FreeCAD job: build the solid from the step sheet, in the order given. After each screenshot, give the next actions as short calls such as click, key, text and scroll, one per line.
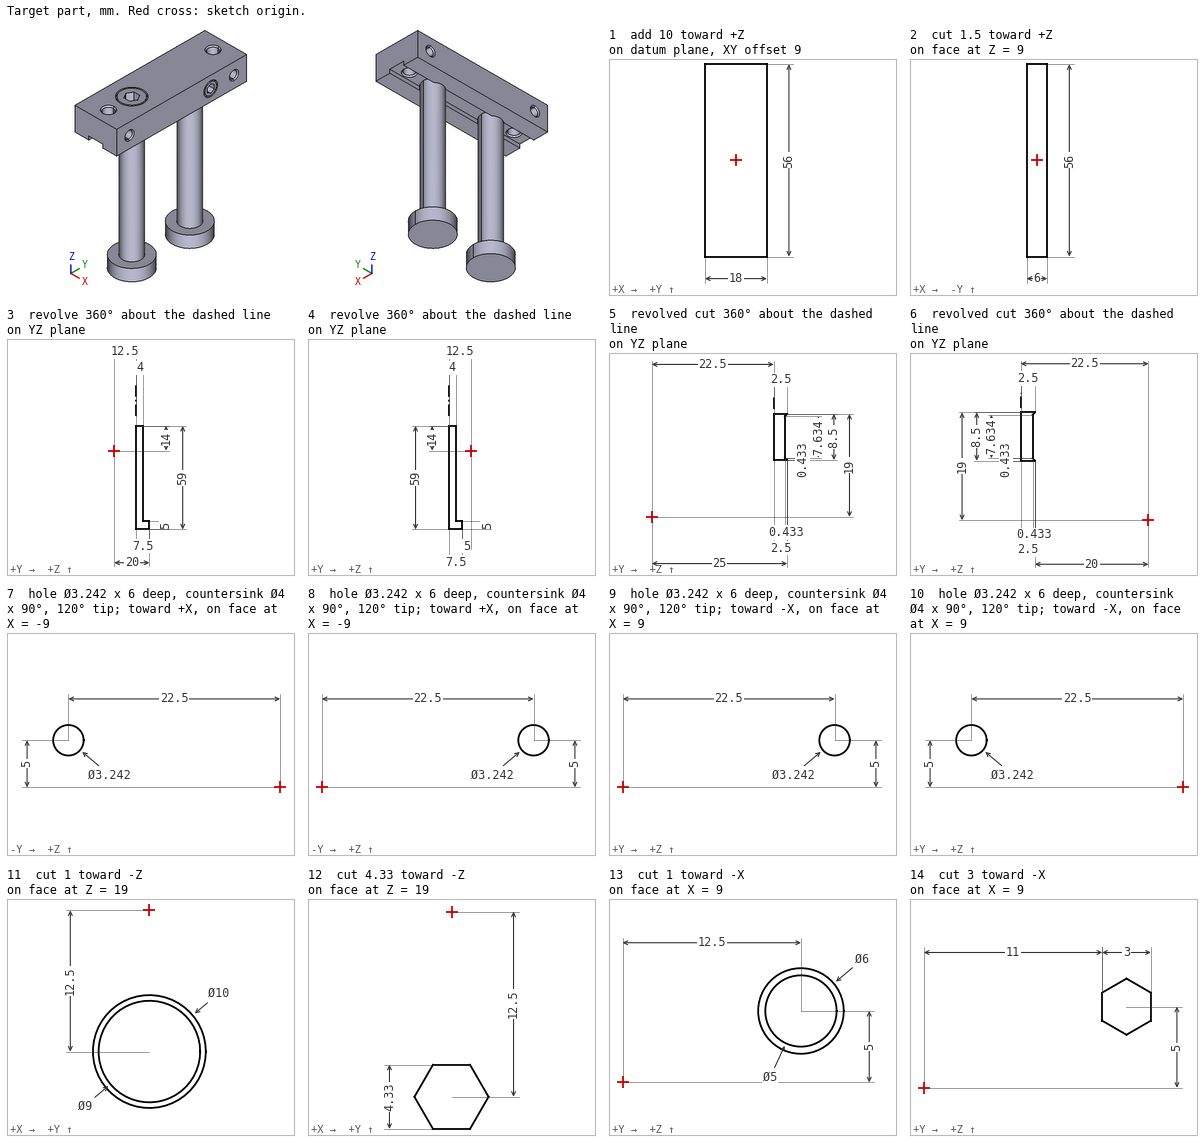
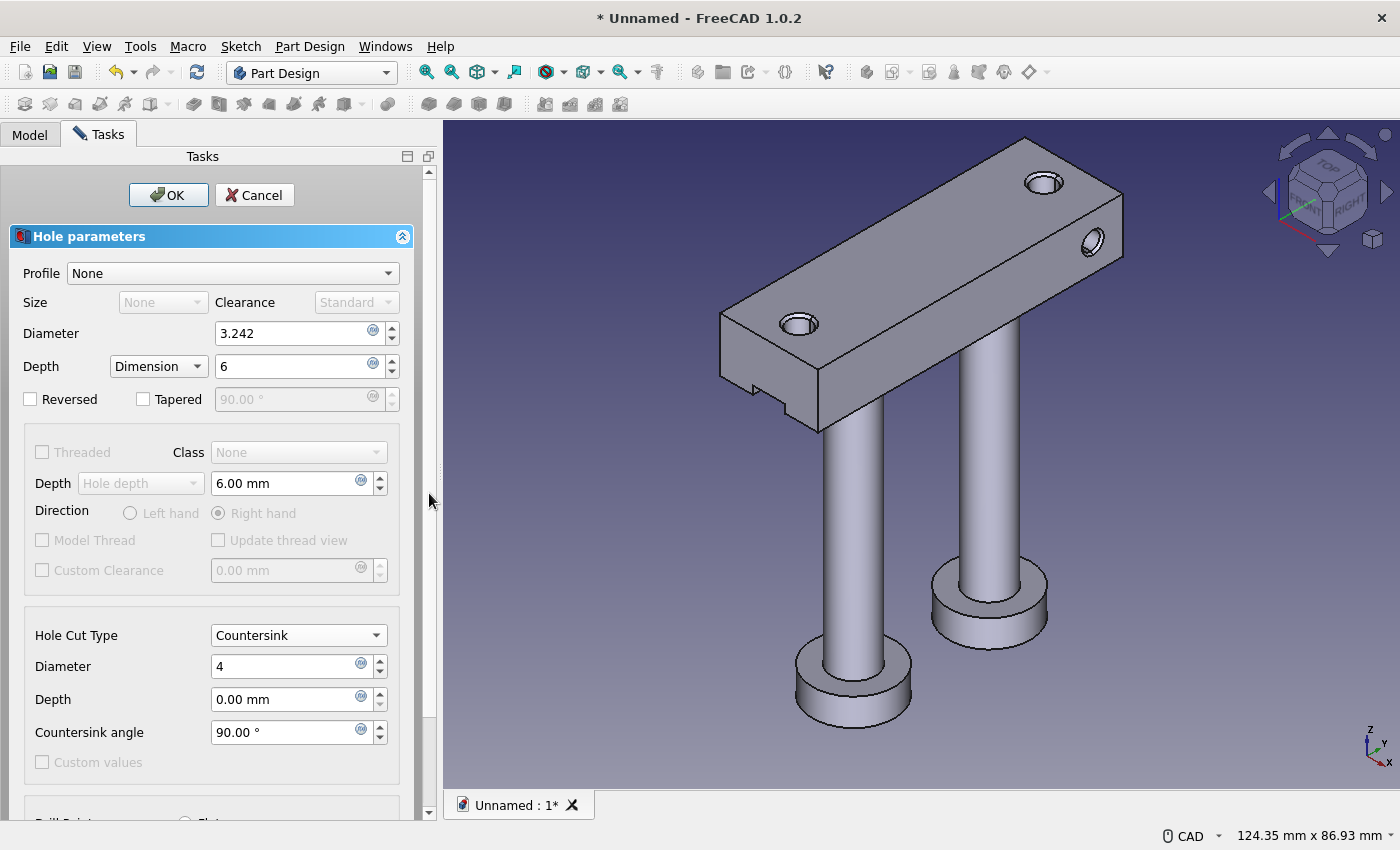
click(169, 195)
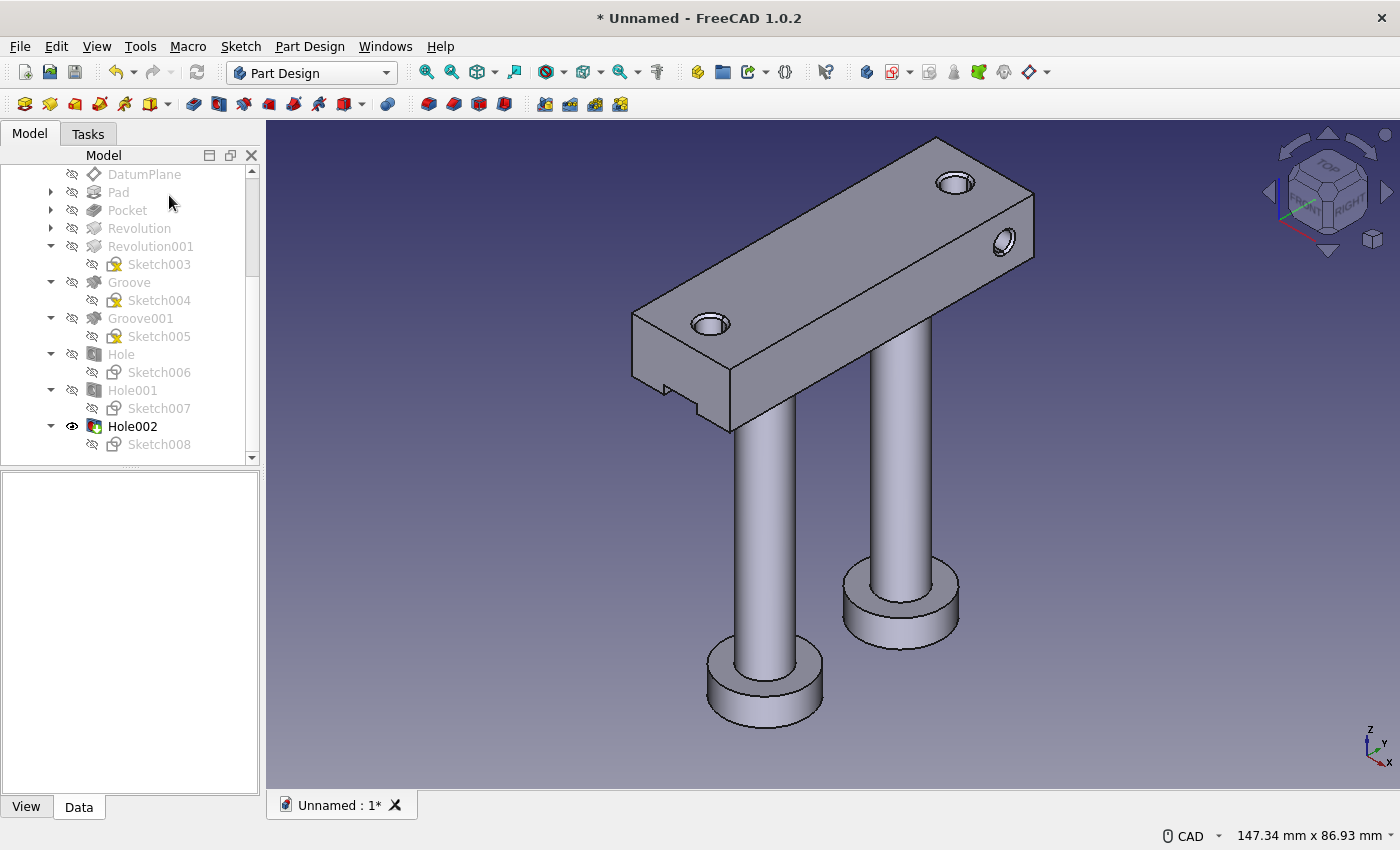
click(926, 287)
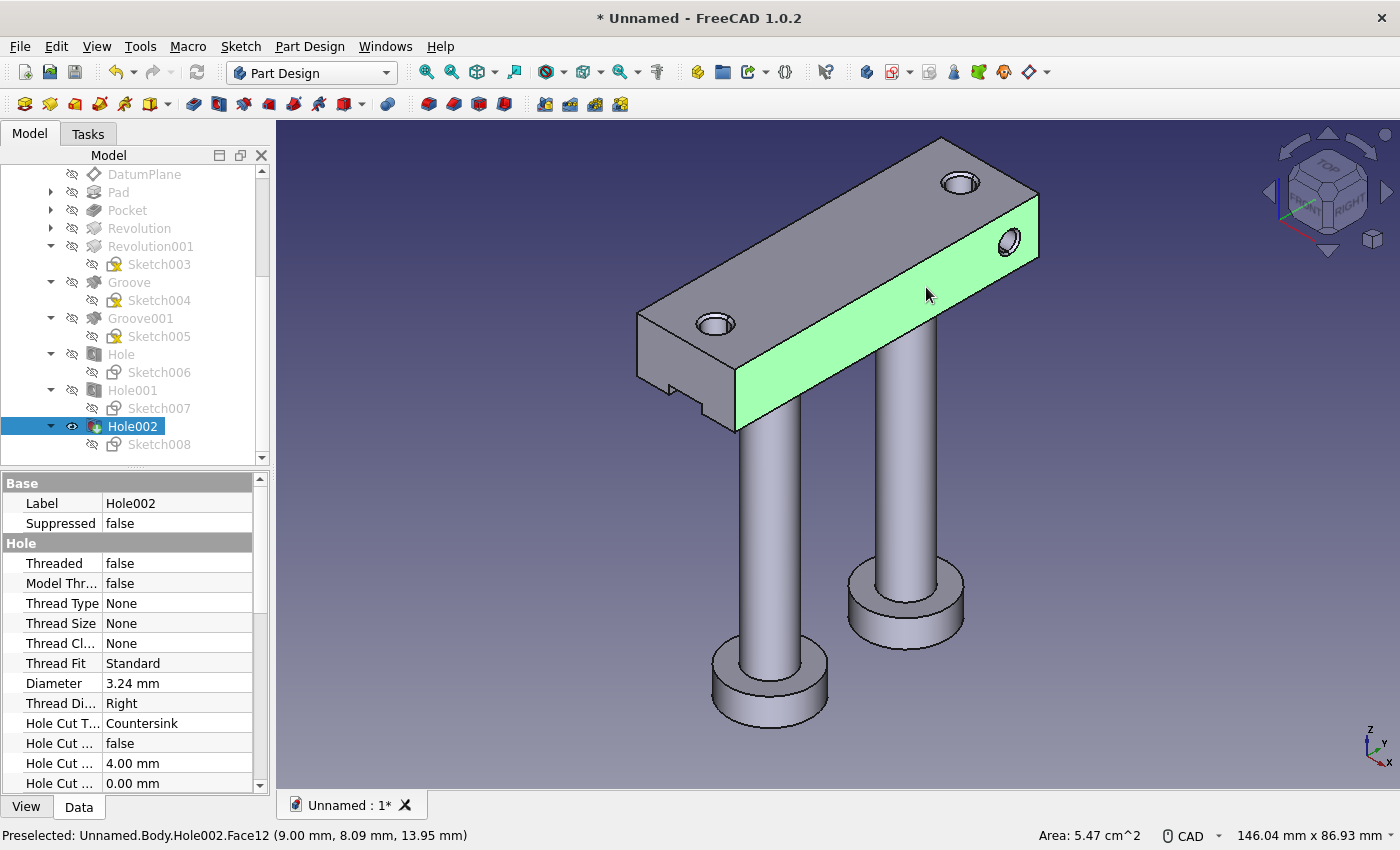
click(892, 72)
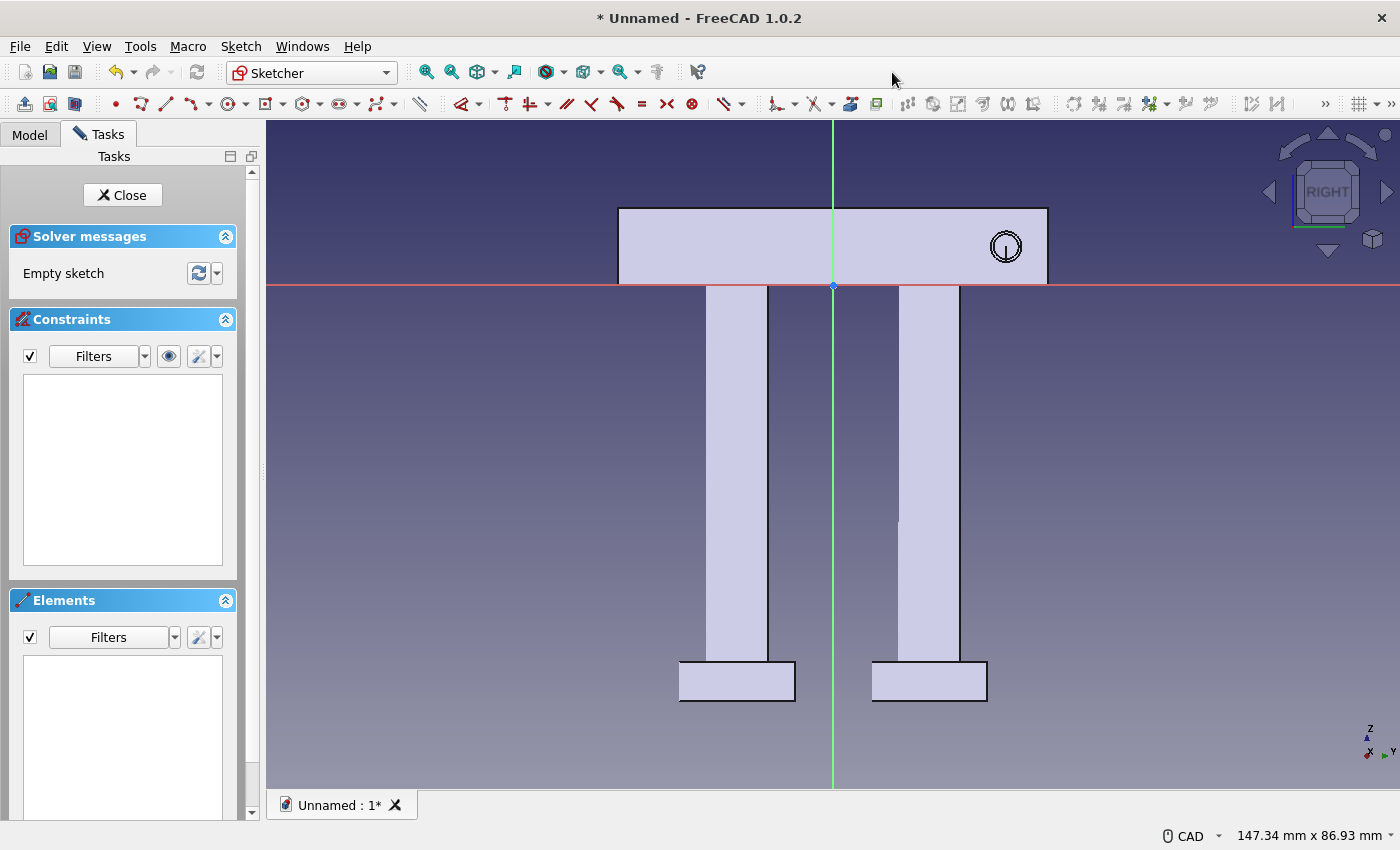
scroll(653, 233, up, 14)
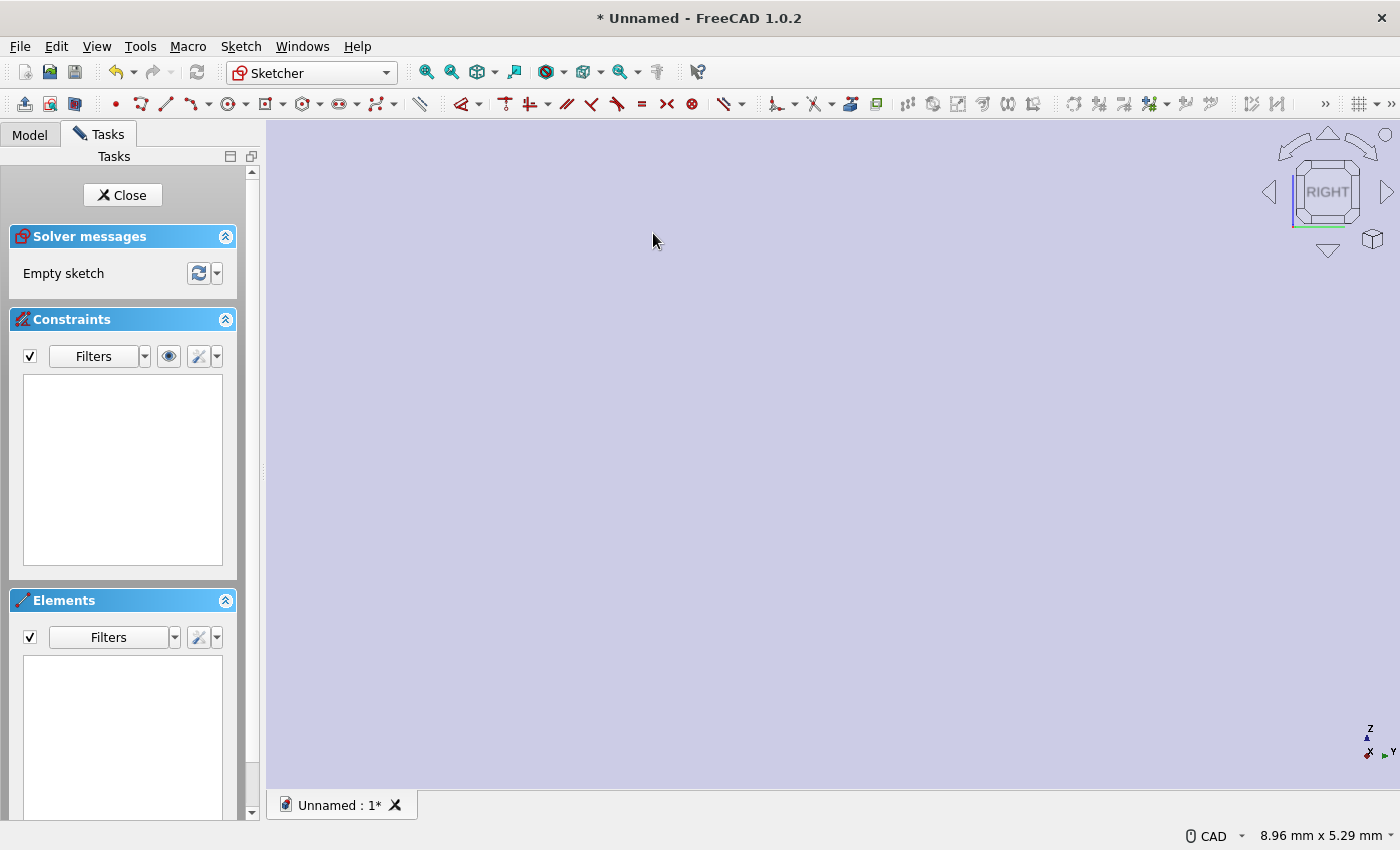
click(228, 104)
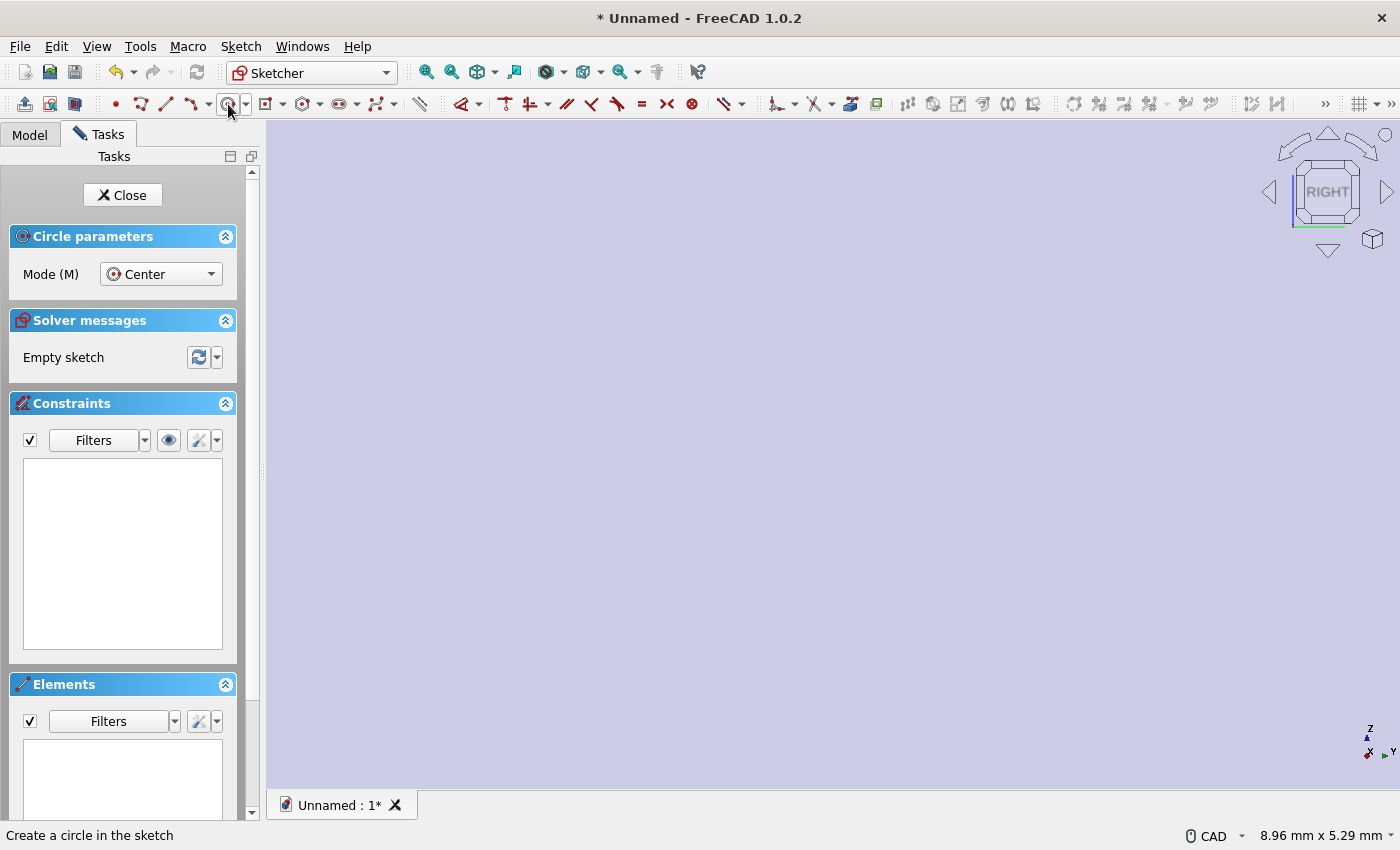
click(760, 456)
move(905, 311)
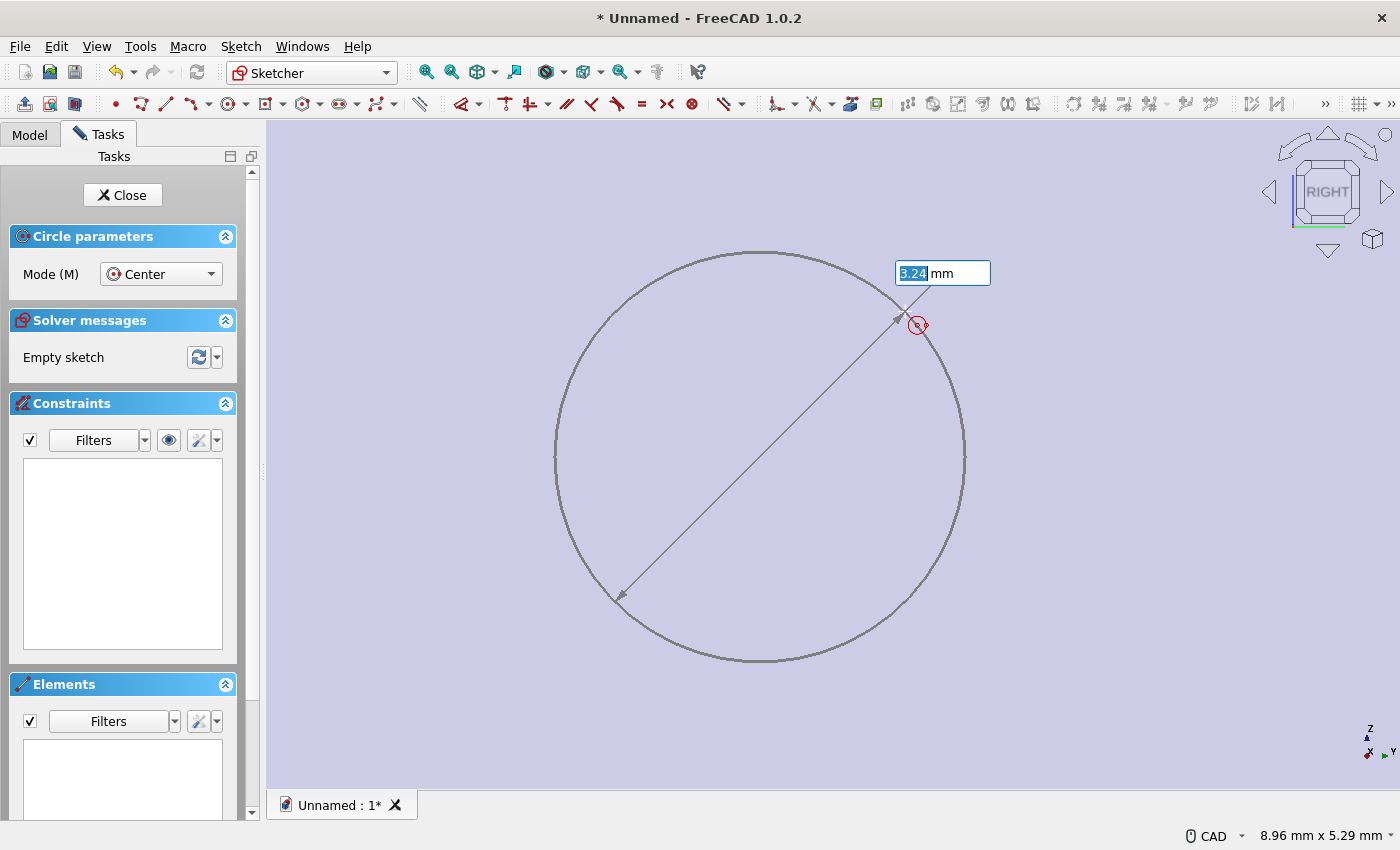
text(3.242)
key(Return)
key(Escape)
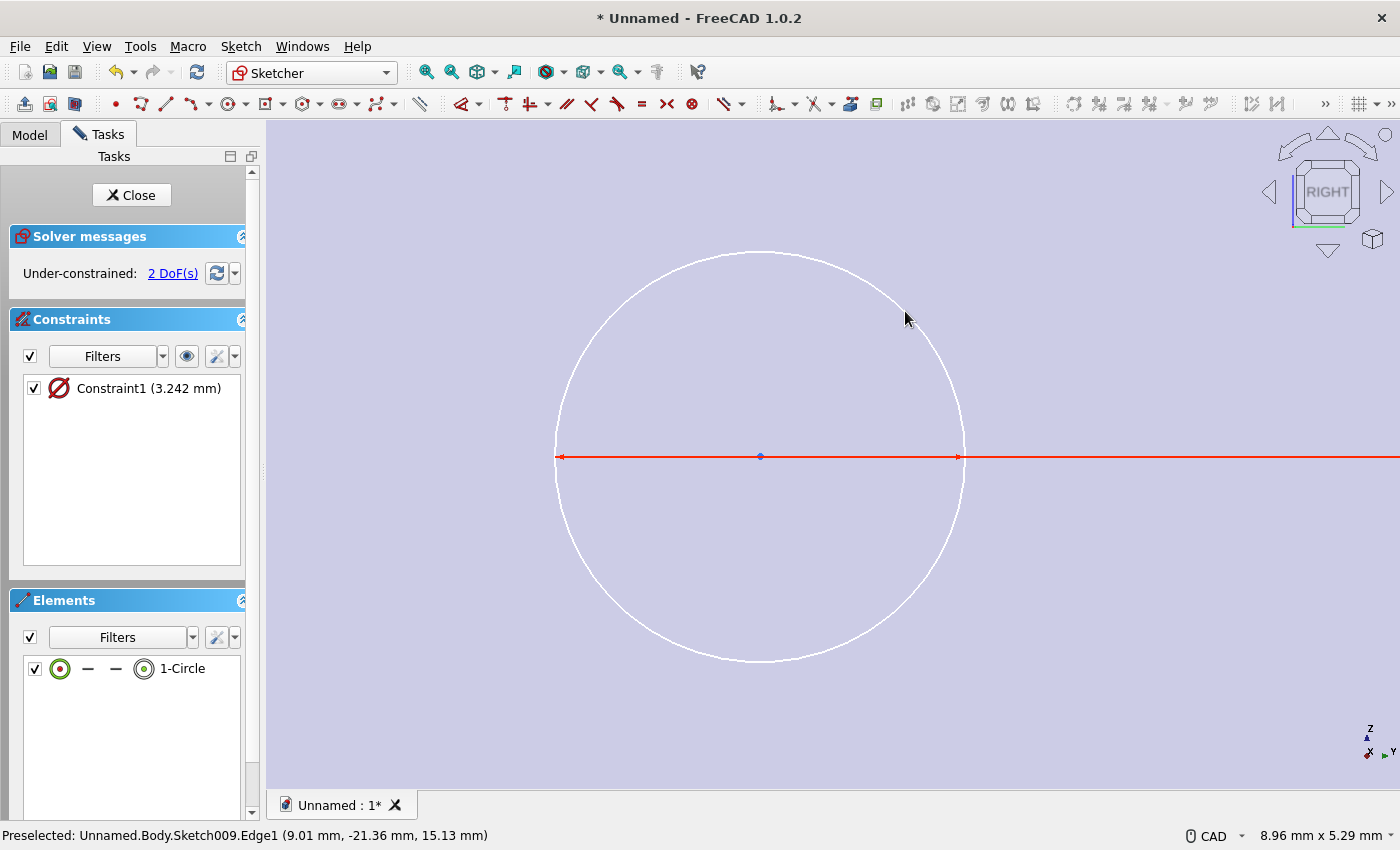
click(460, 104)